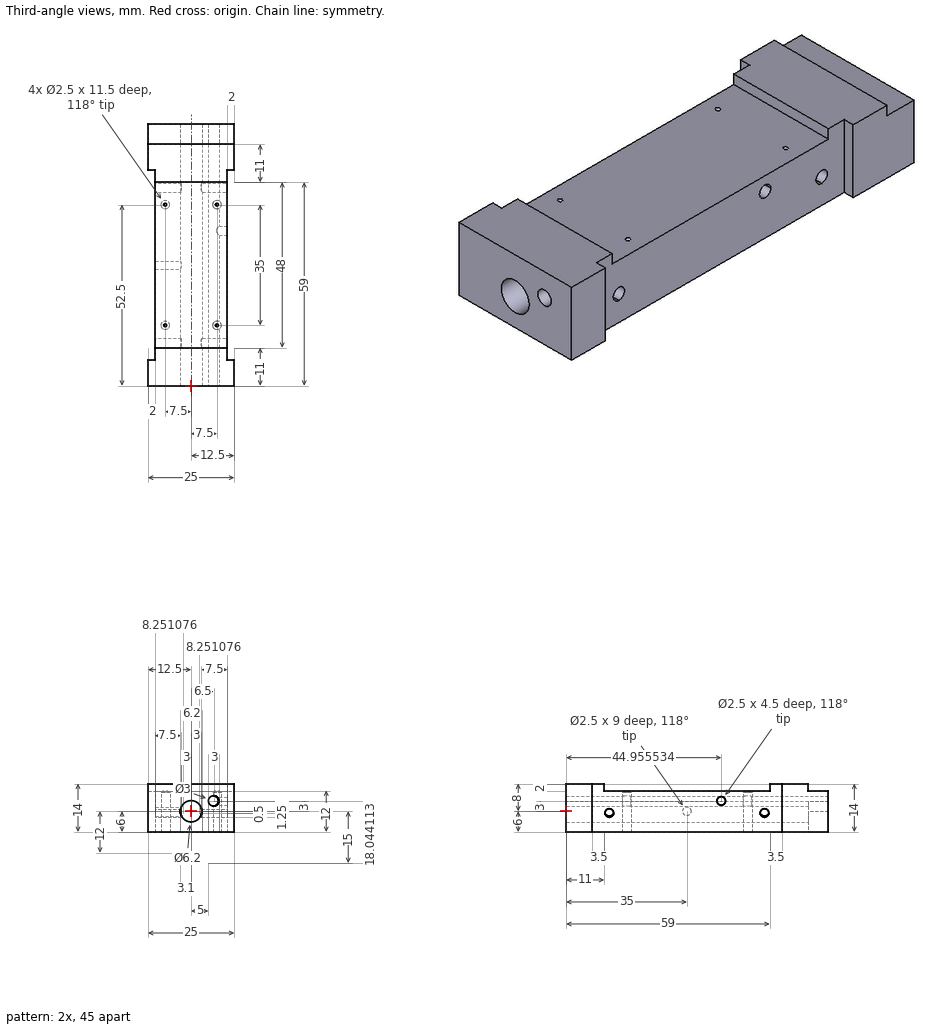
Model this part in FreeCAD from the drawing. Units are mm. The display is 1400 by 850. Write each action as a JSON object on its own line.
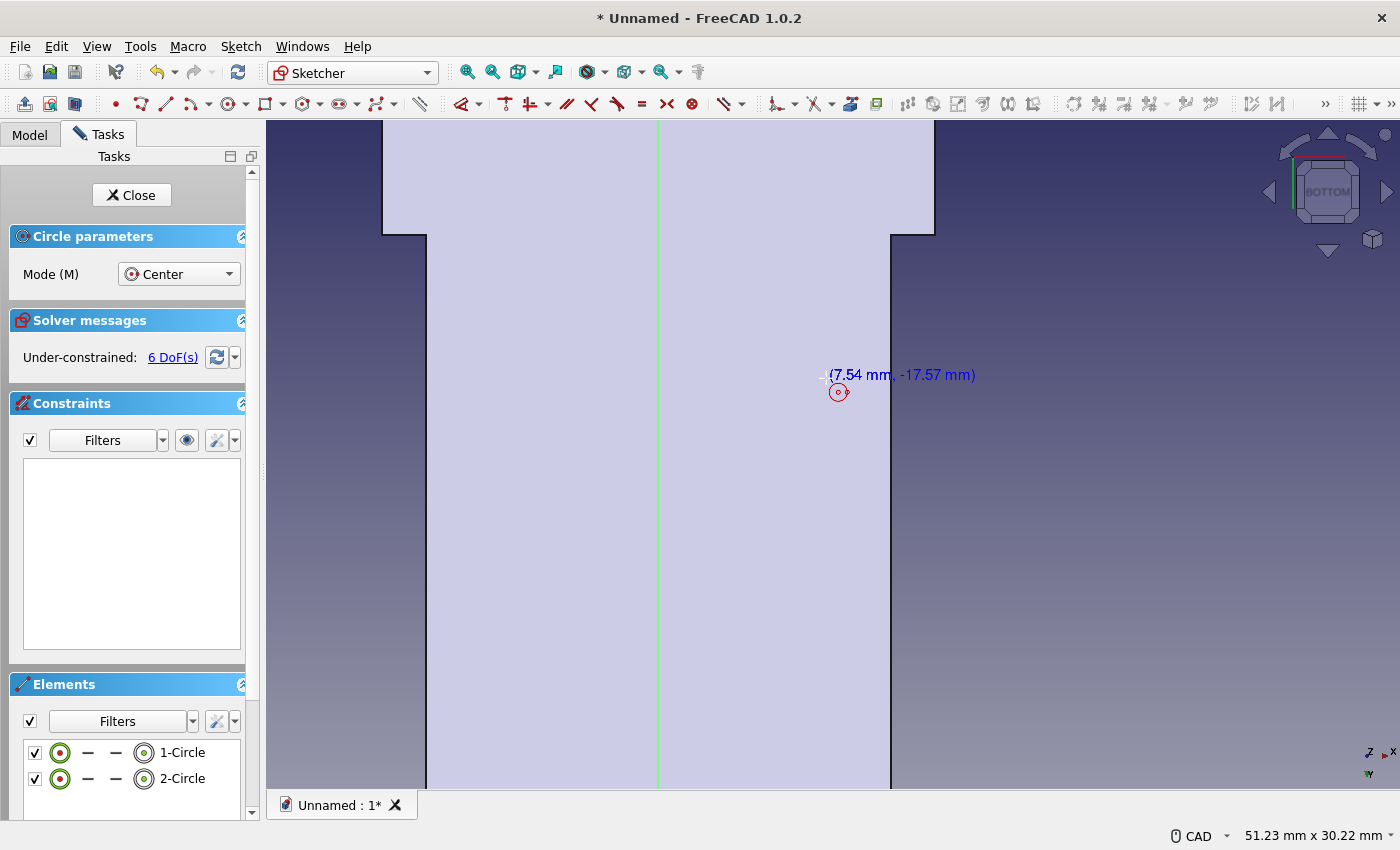
{"action": "left_click", "coordinate": [824, 379]}
{"action": "left_click", "coordinate": [844, 359]}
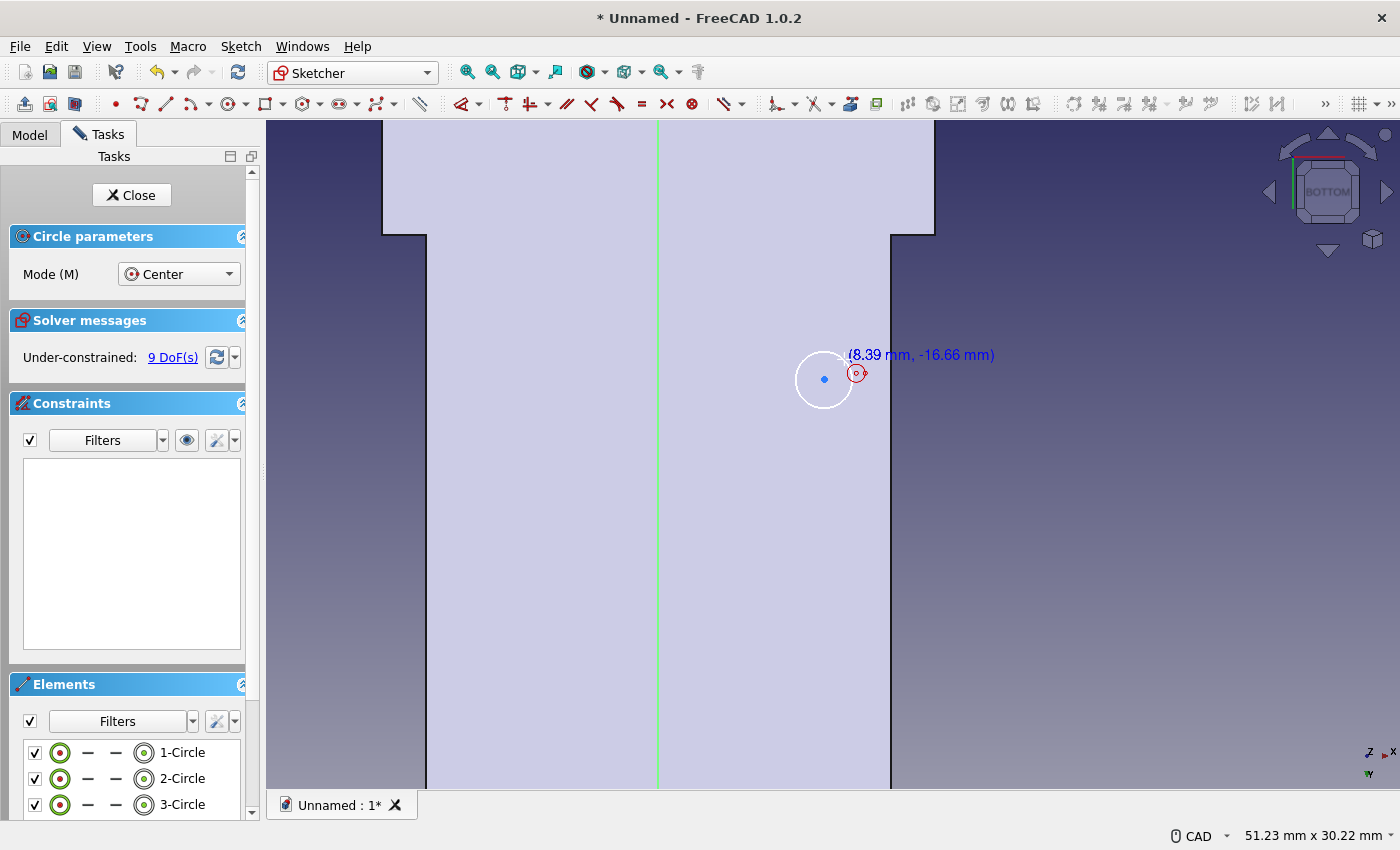
{"action": "left_click", "coordinate": [492, 379]}
{"action": "left_click", "coordinate": [512, 359]}
{"action": "key", "text": "Escape"}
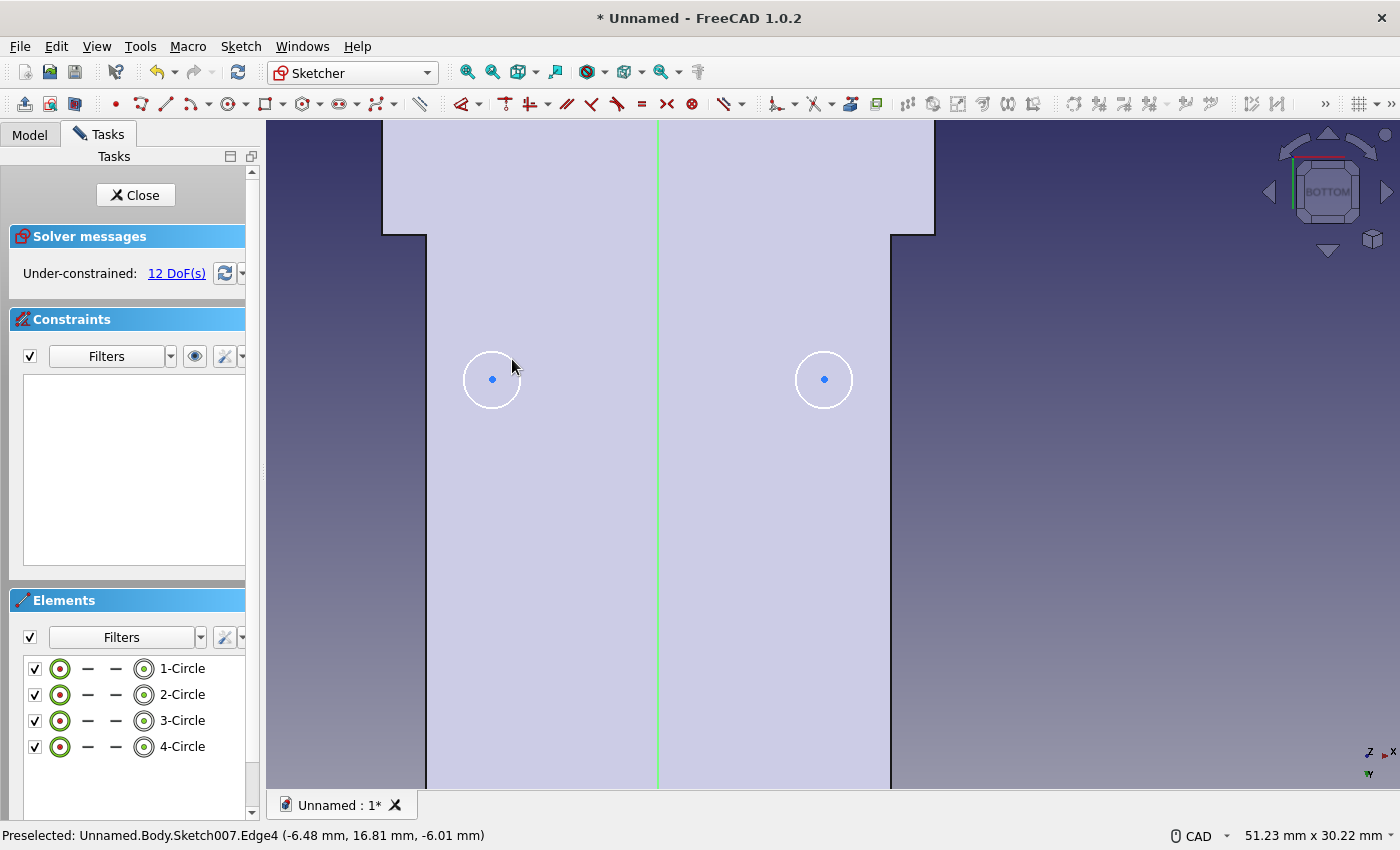
{"action": "scroll", "coordinate": [826, 378], "scroll_direction": "down", "scroll_amount": 5}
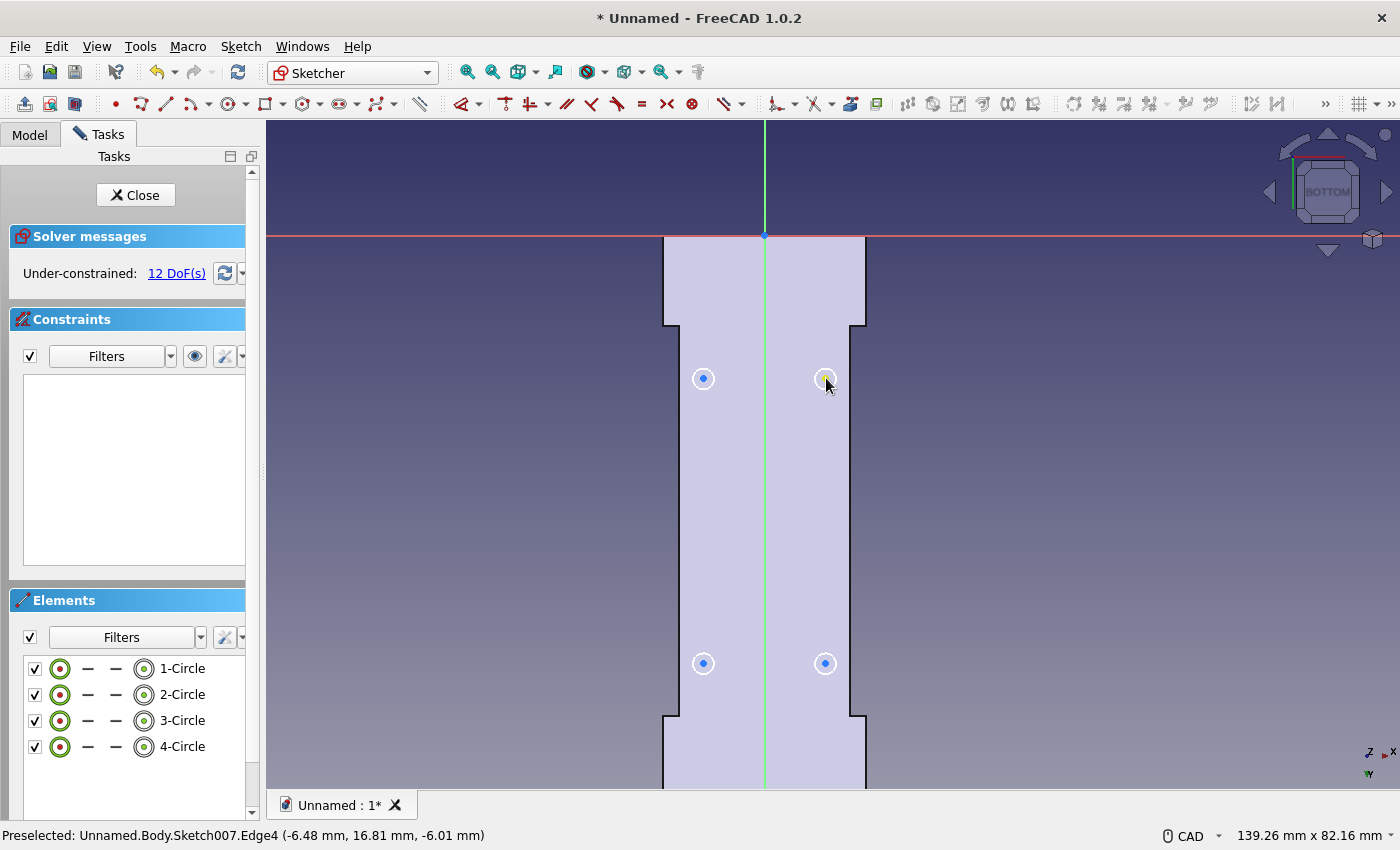
{"action": "scroll", "coordinate": [711, 656], "scroll_direction": "up", "scroll_amount": 2}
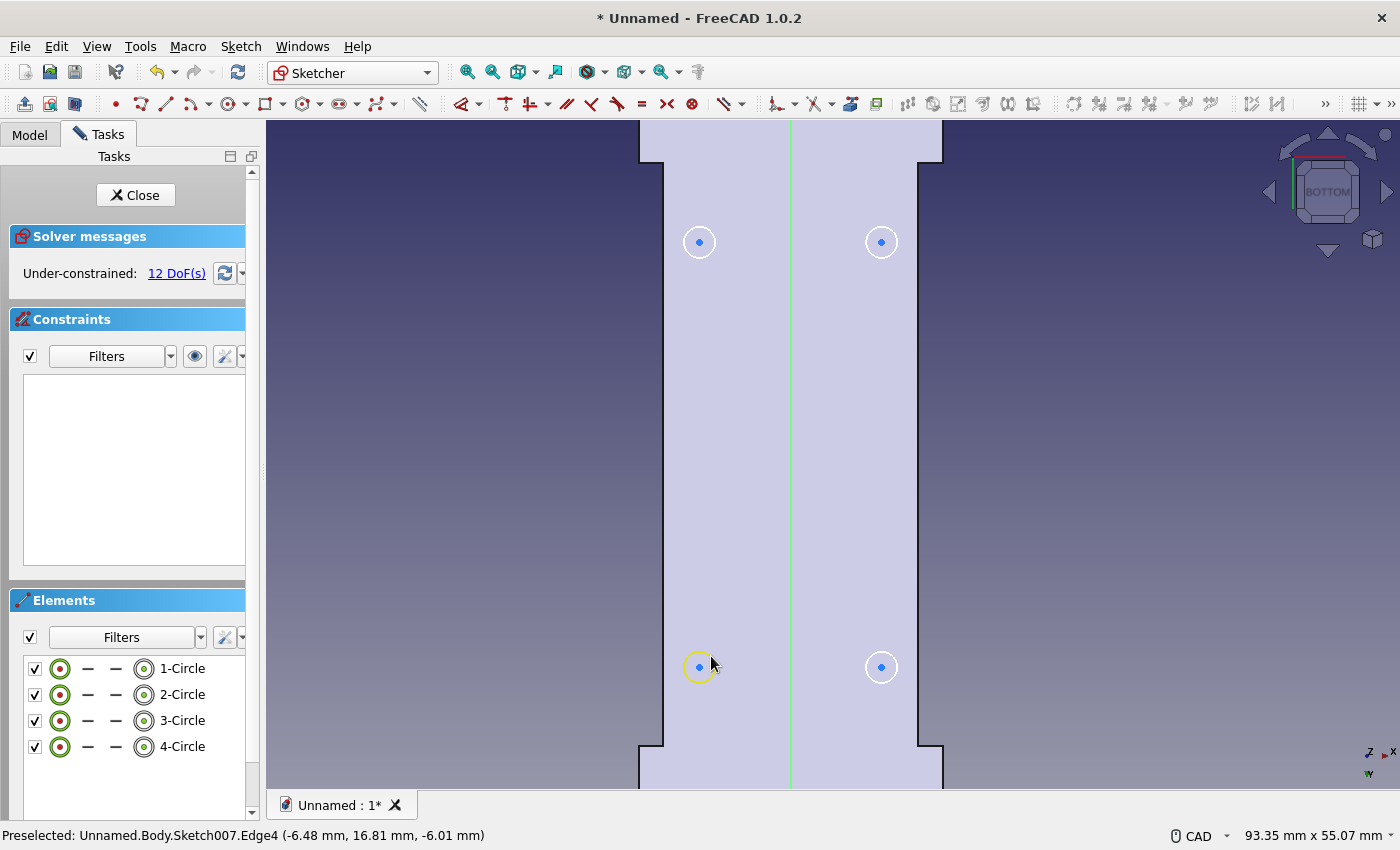
{"action": "left_click", "coordinate": [710, 656]}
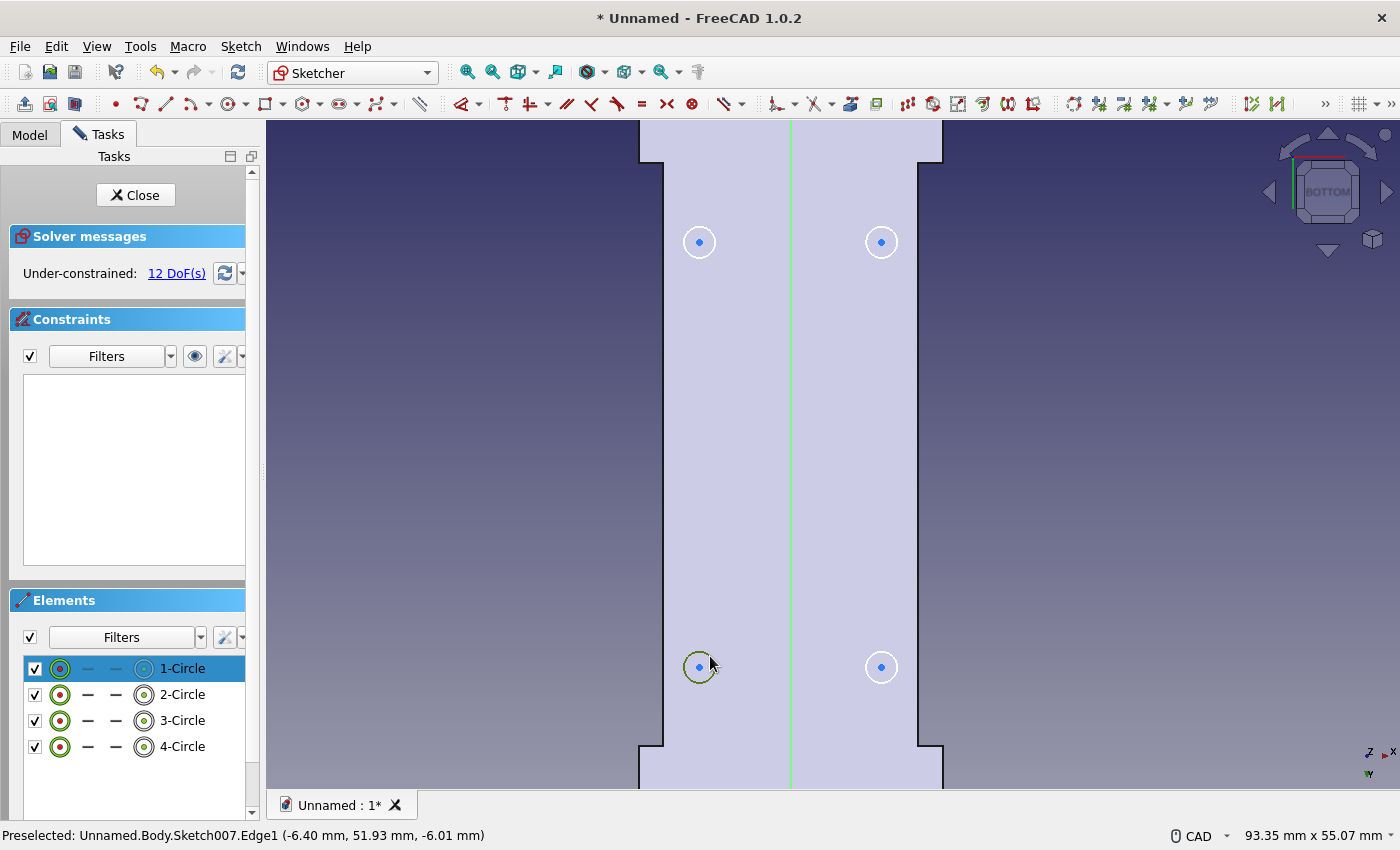
{"action": "left_click", "coordinate": [893, 656]}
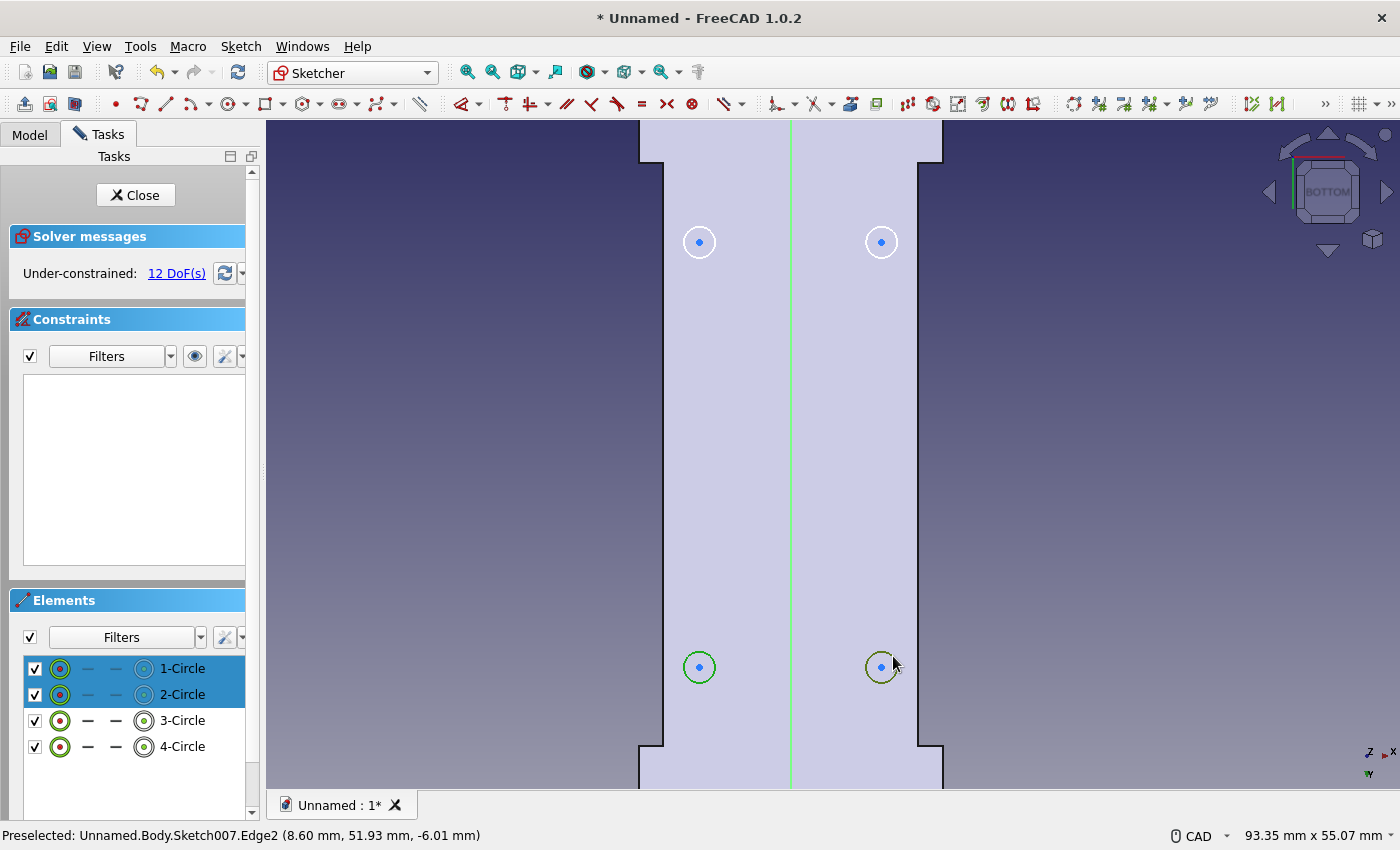
{"action": "left_click", "coordinate": [893, 231]}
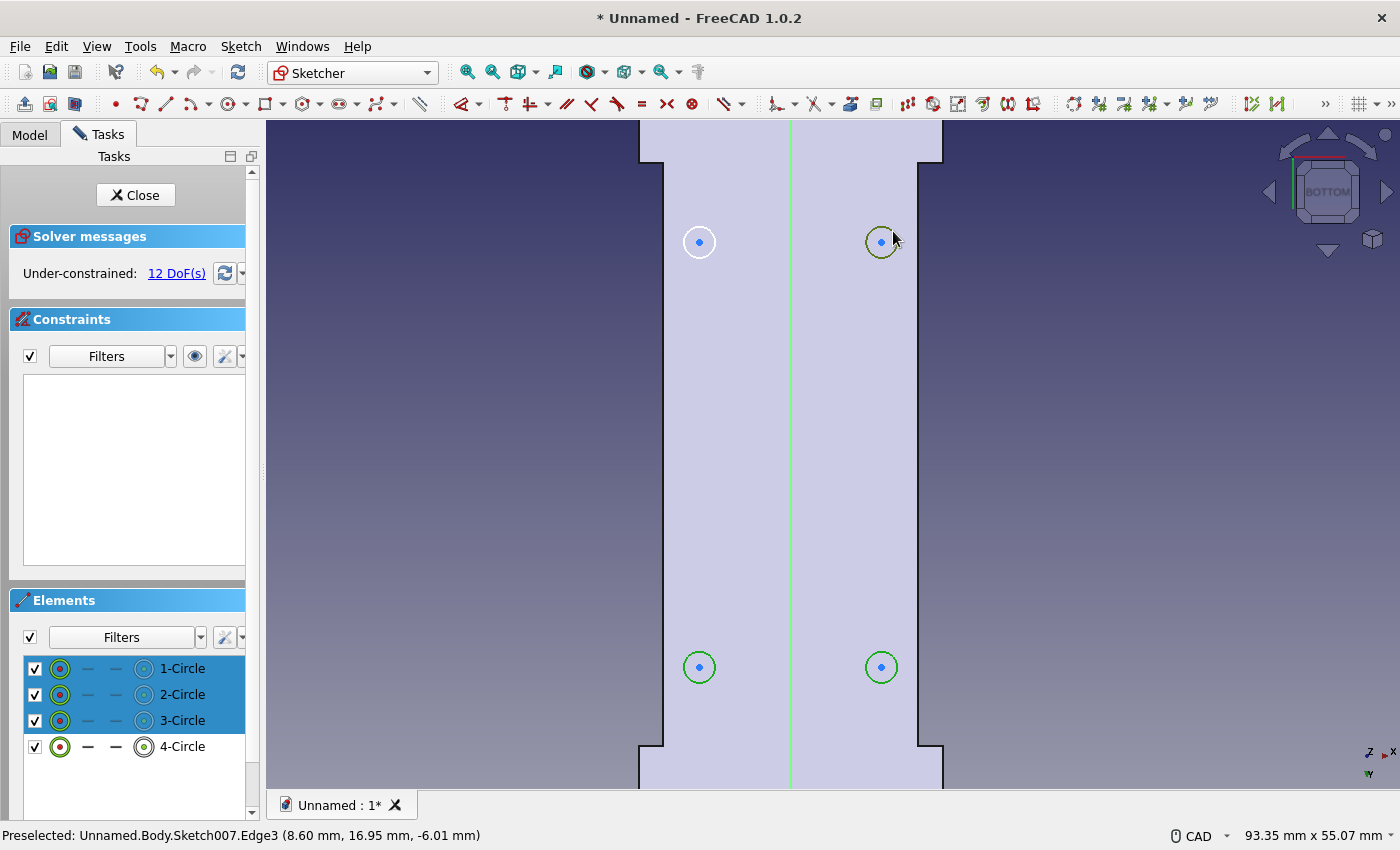
{"action": "left_click", "coordinate": [710, 231]}